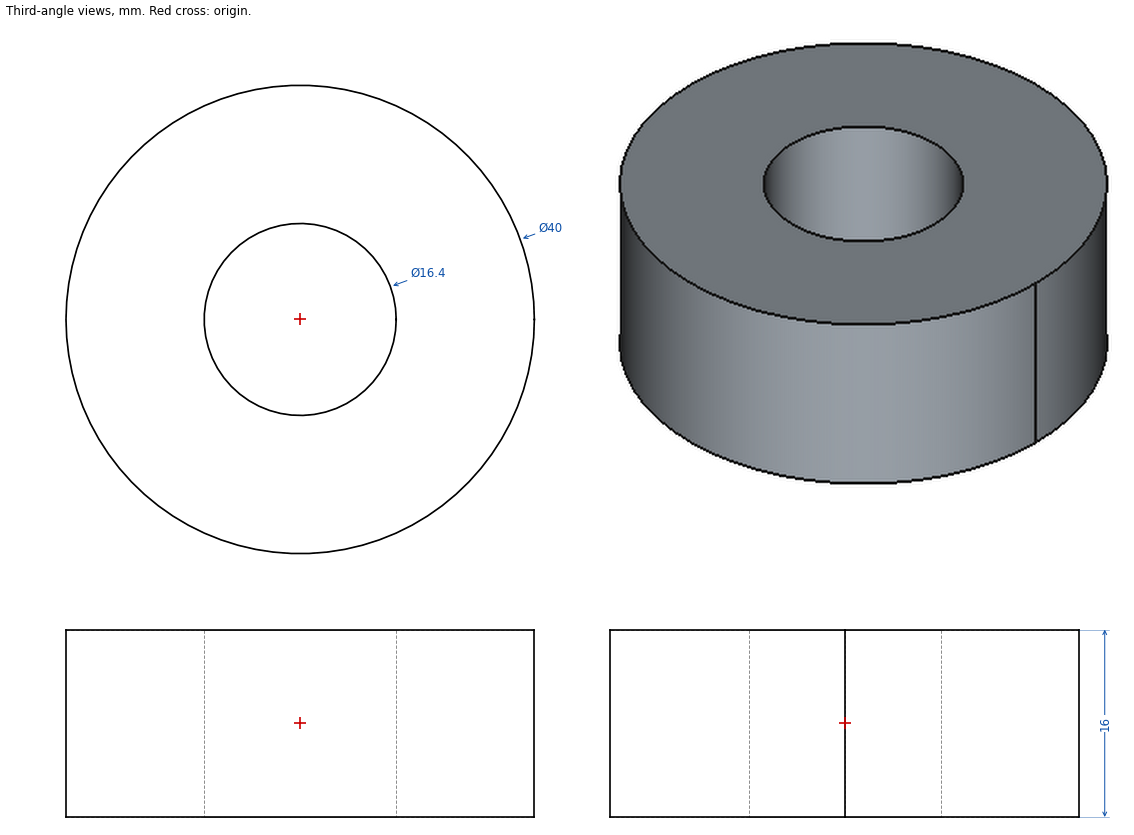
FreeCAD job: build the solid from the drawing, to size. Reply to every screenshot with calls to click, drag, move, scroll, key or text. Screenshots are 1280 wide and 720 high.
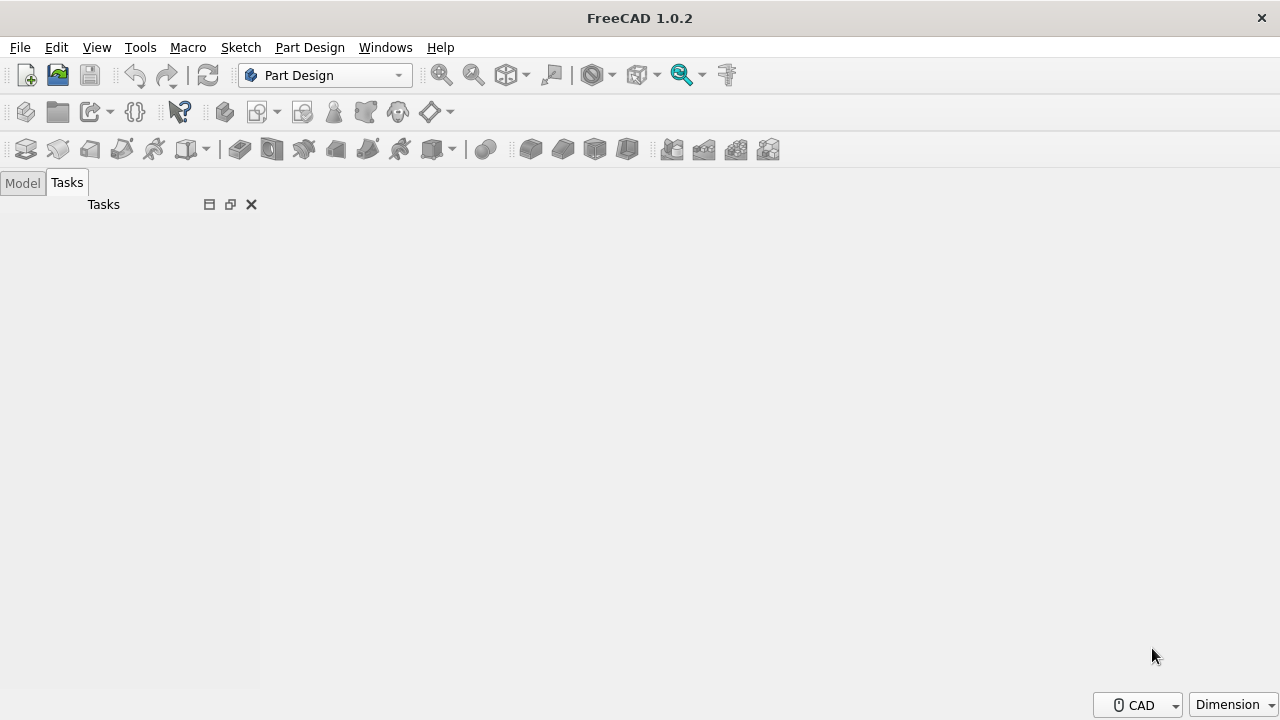
click(26, 76)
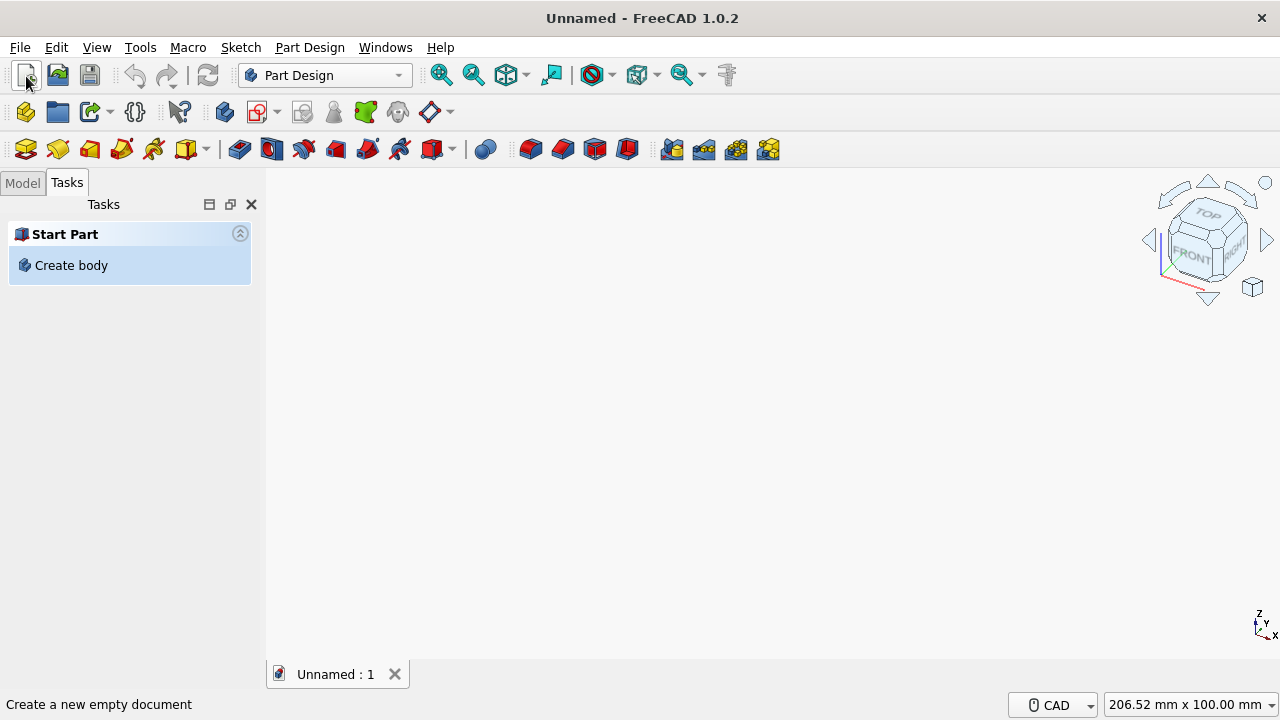
click(258, 112)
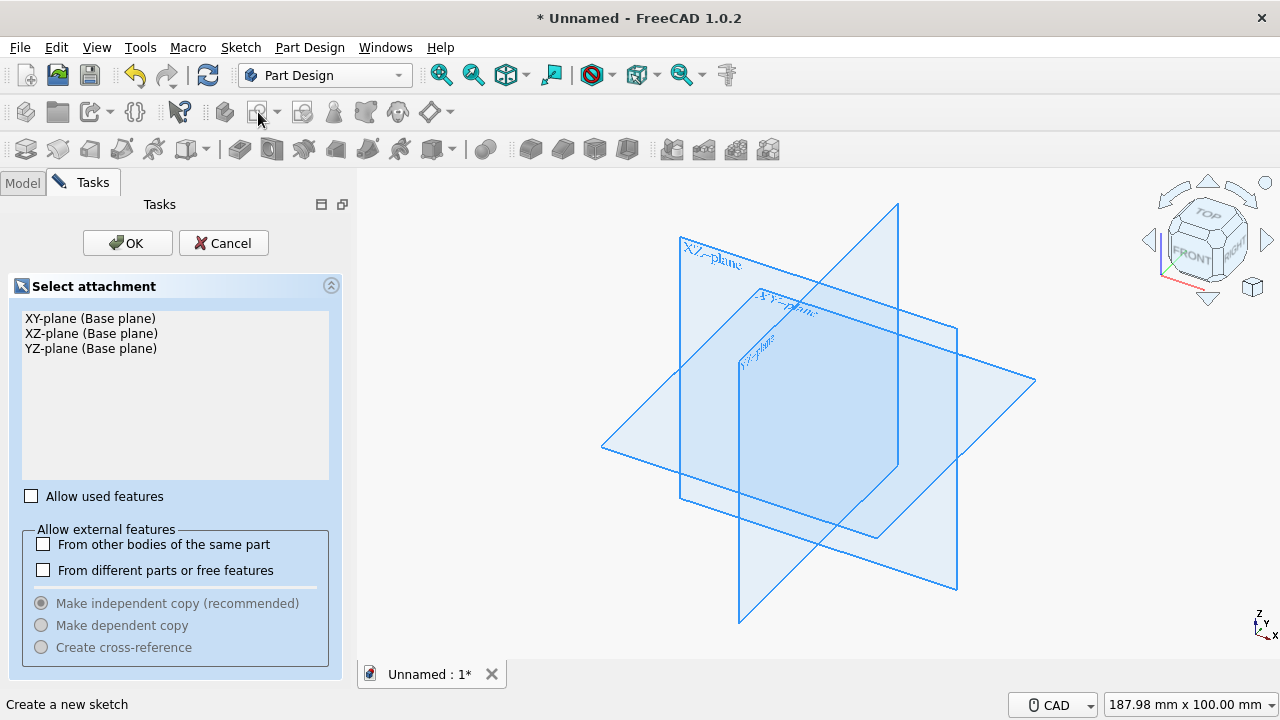
click(82, 318)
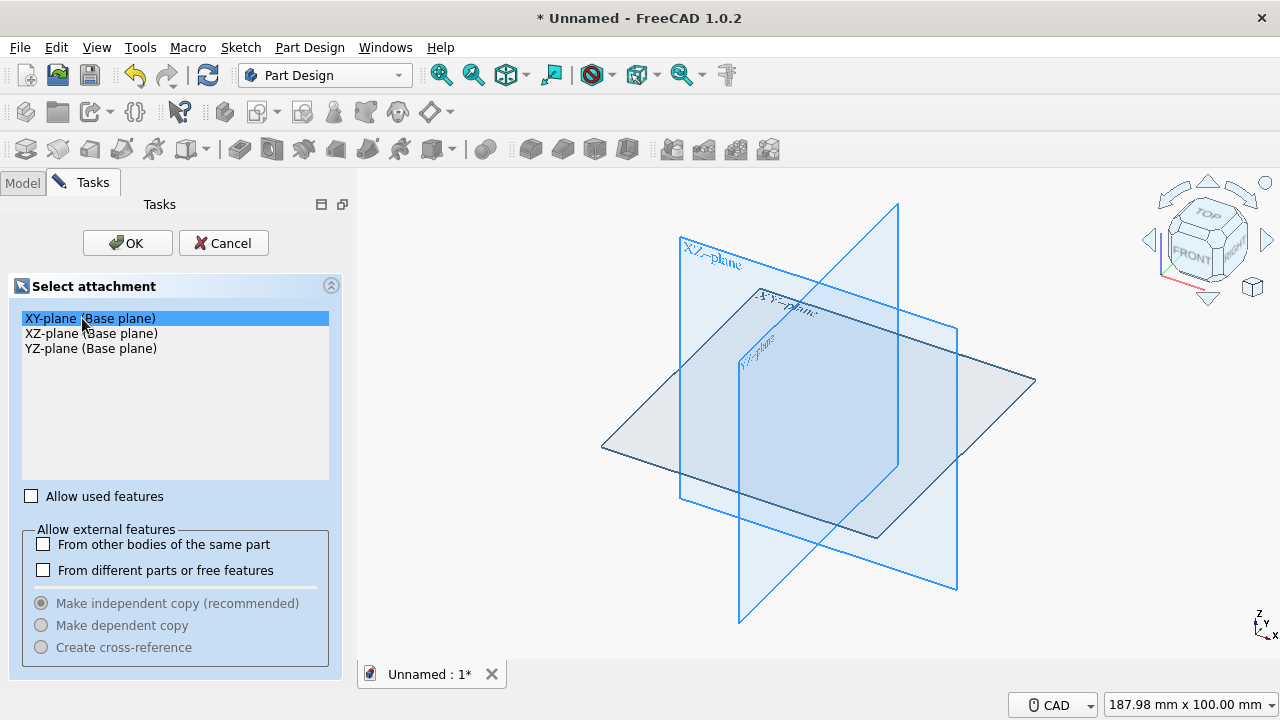
click(128, 243)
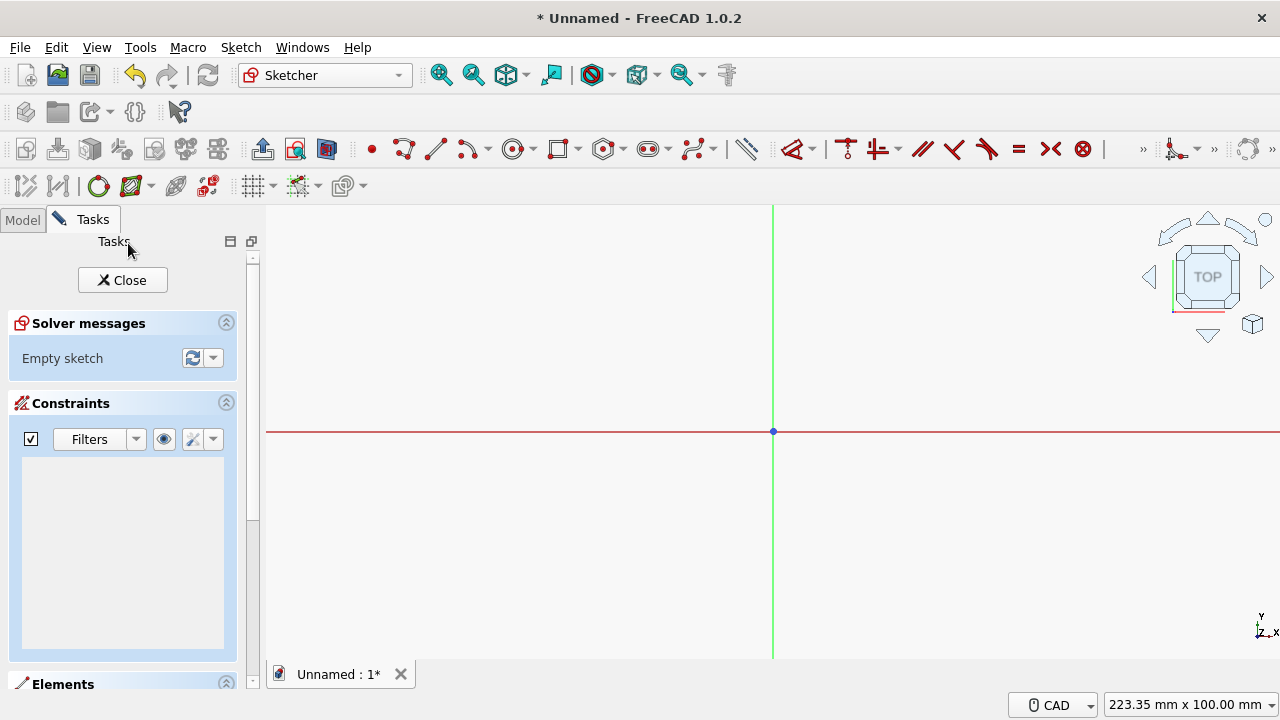
scroll(912, 432, up, 2)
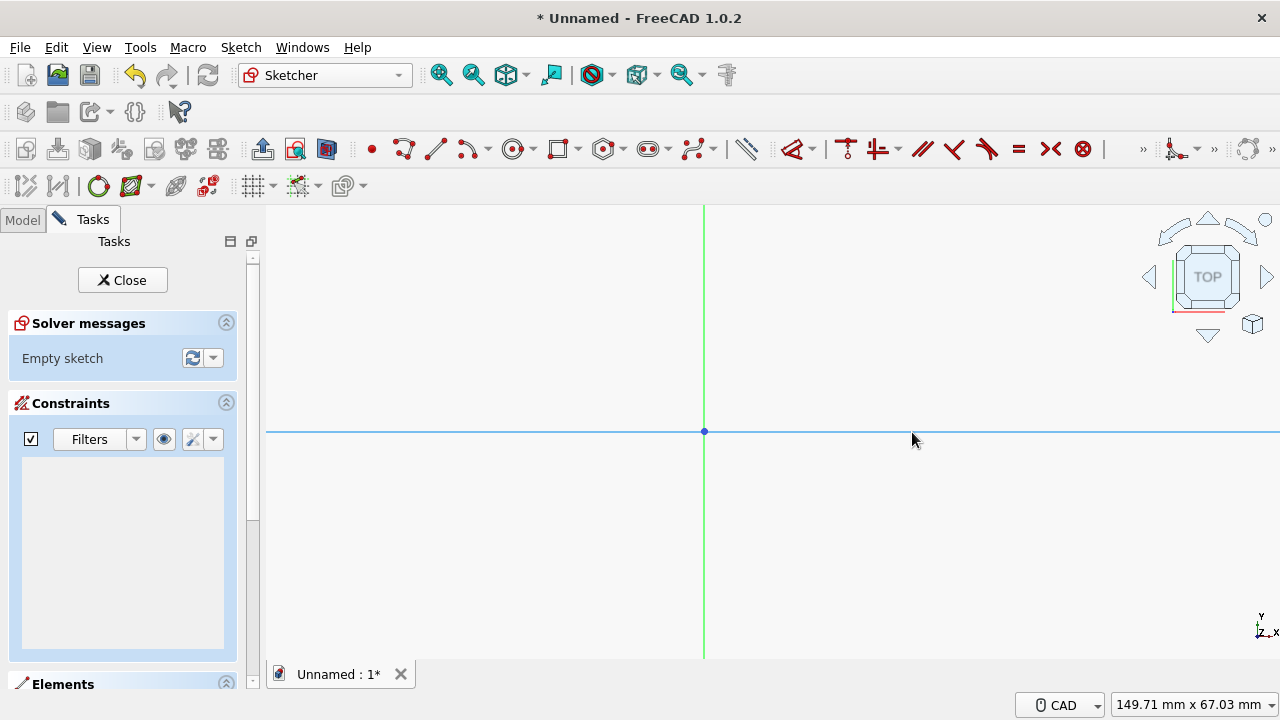
click(514, 150)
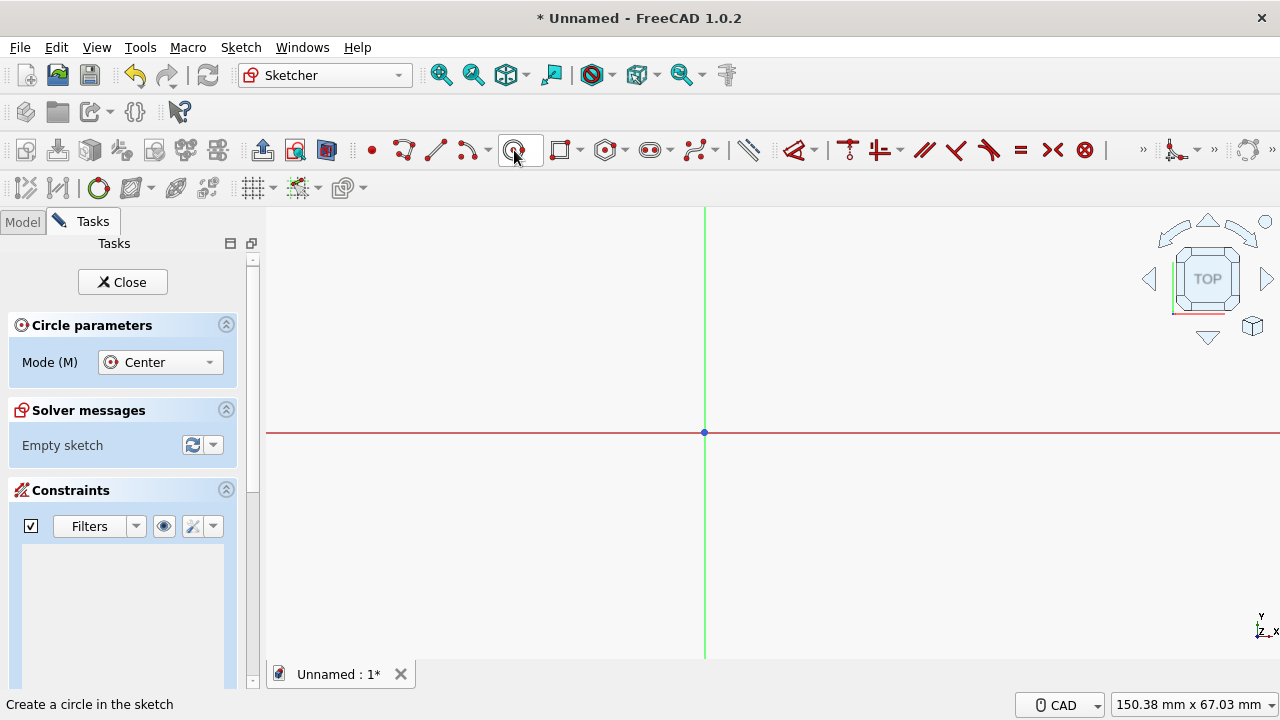
click(705, 433)
move(800, 337)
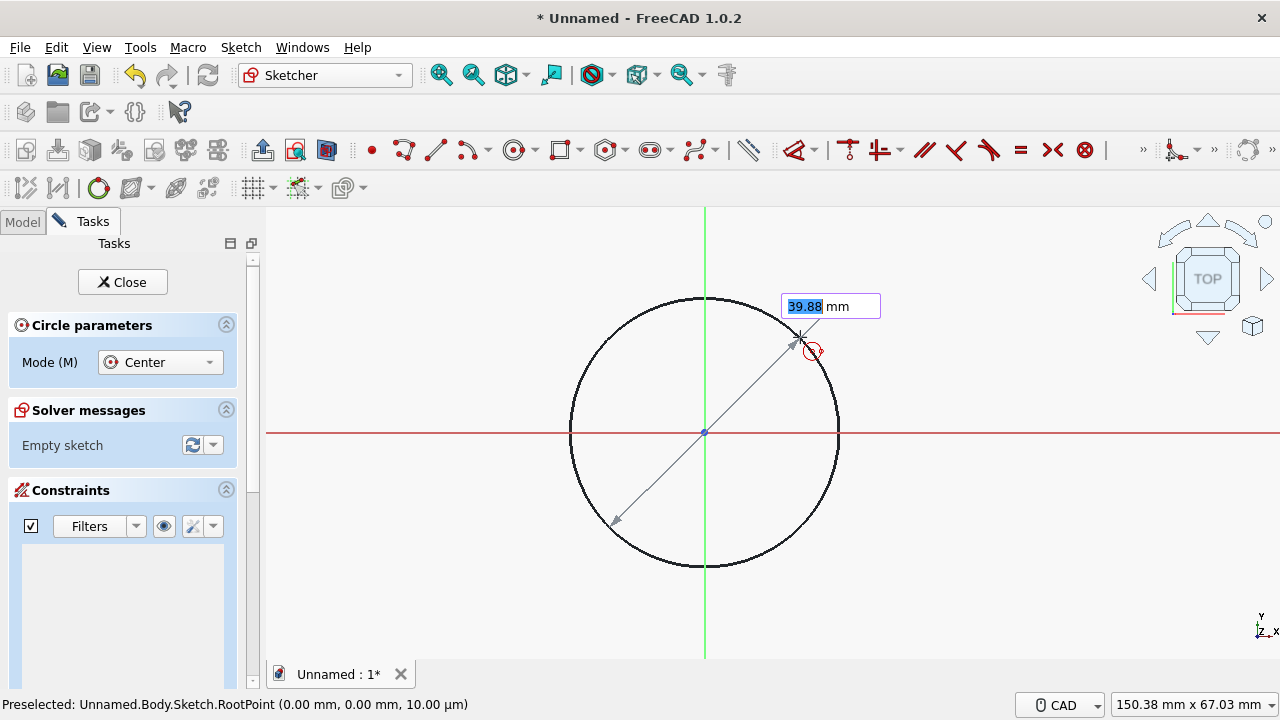
text(40)
key(Return)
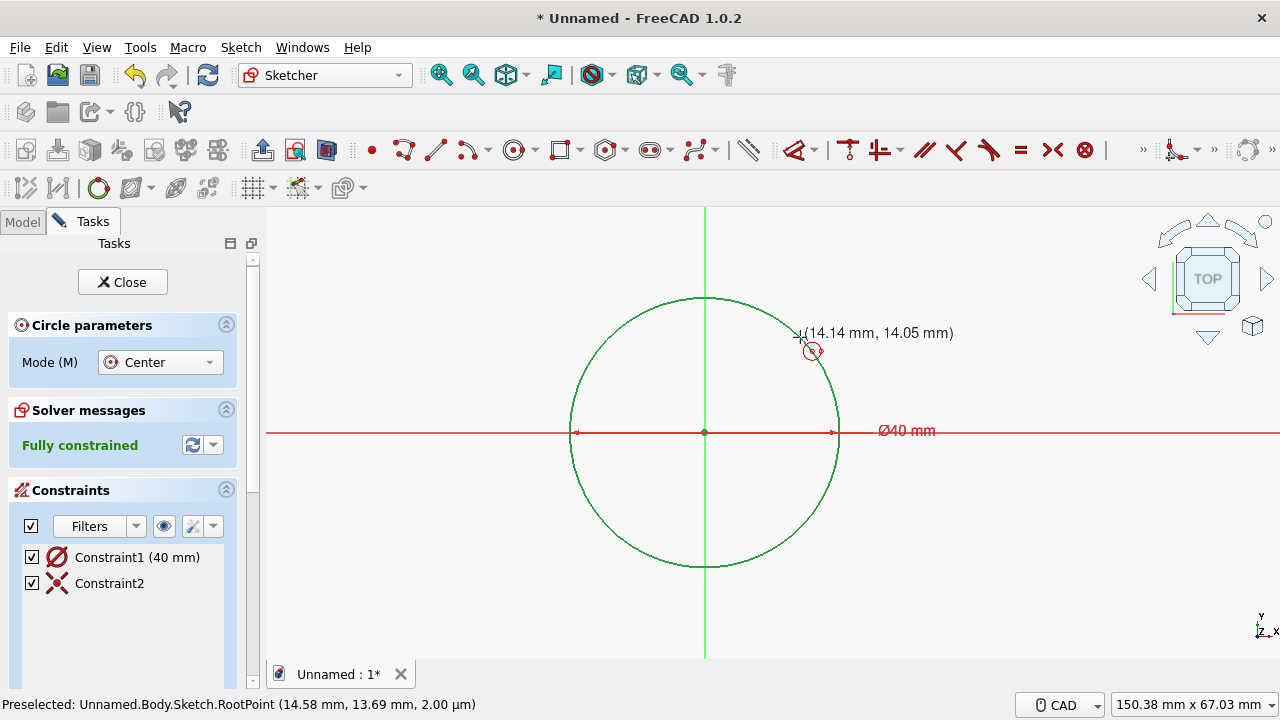
click(705, 433)
move(744, 394)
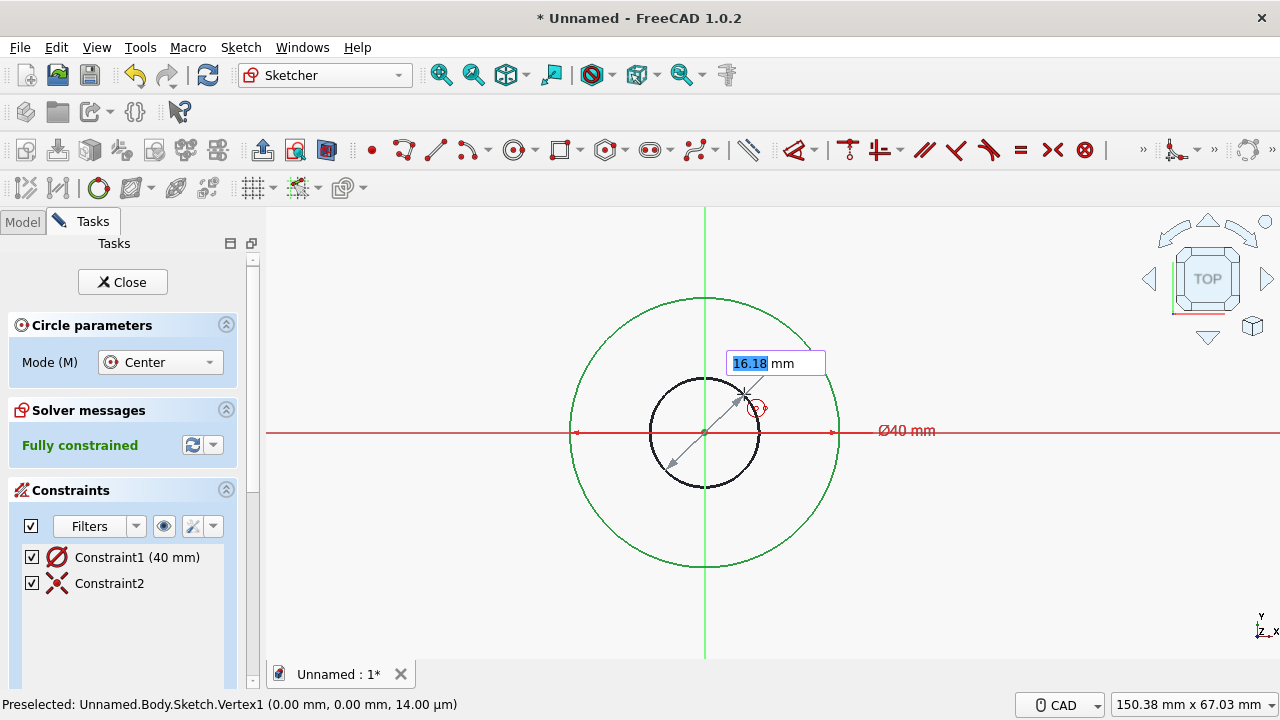
text(16.4)
key(Return)
key(Escape)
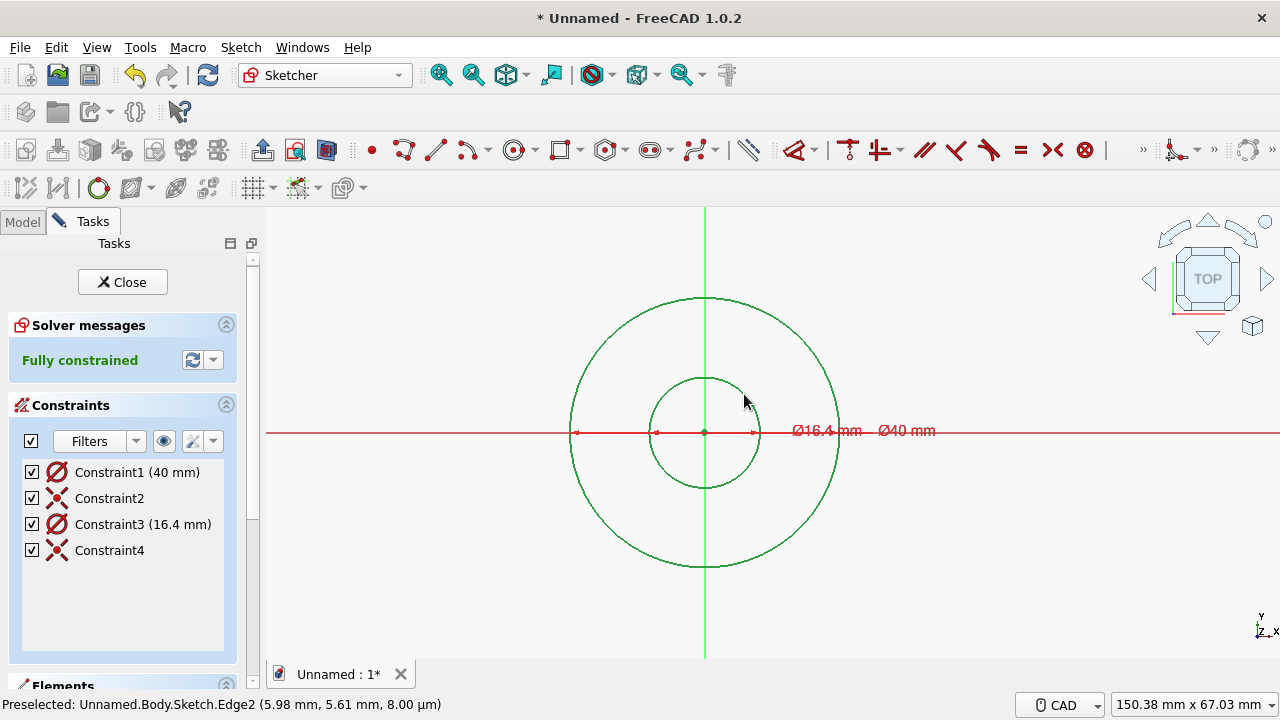
click(123, 282)